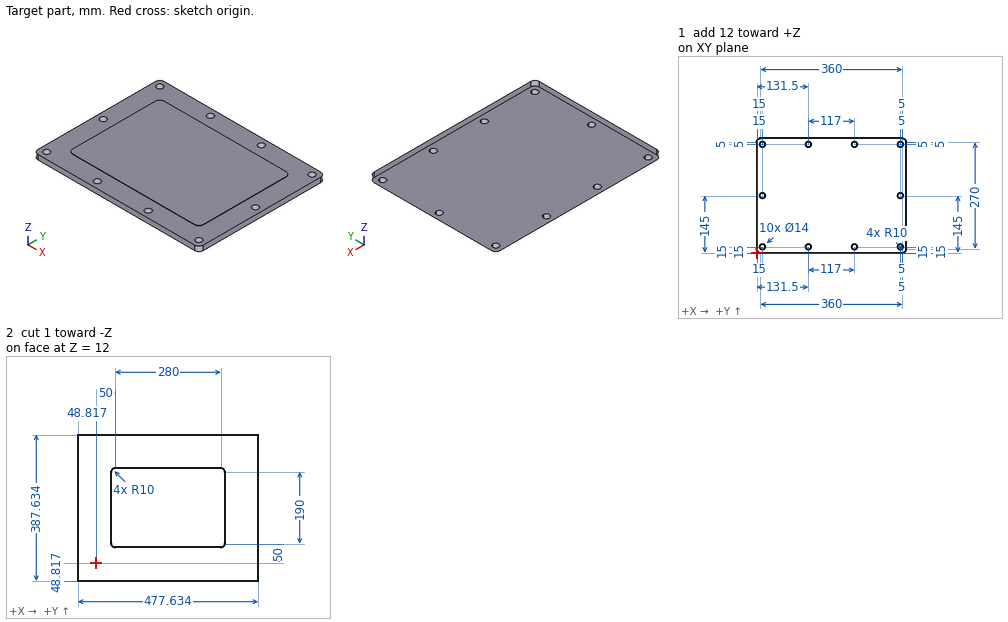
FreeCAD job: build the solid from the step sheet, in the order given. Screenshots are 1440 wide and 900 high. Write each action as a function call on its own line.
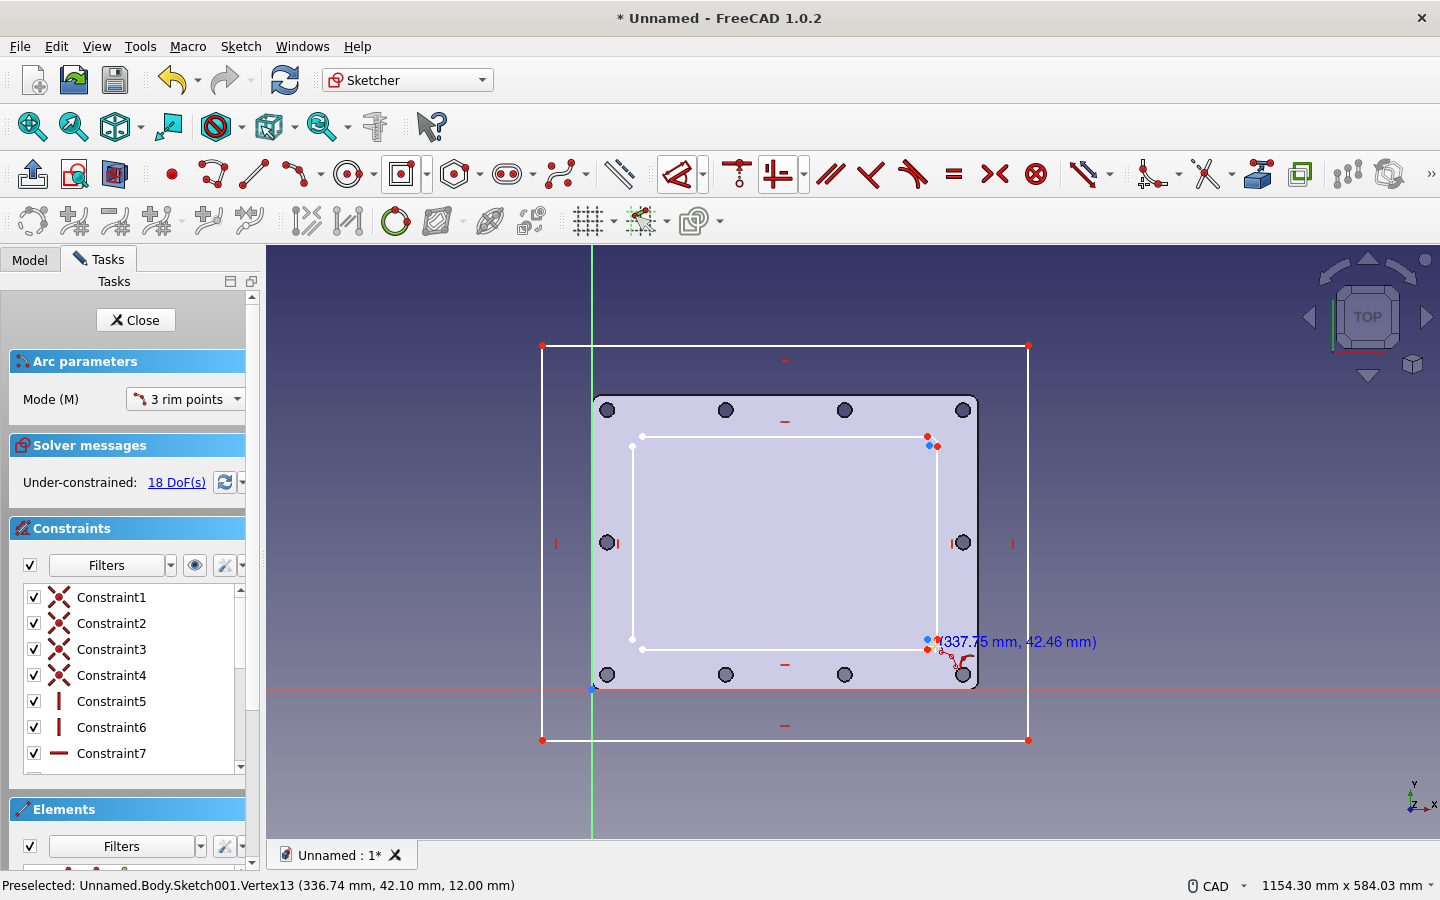
click(643, 650)
click(633, 640)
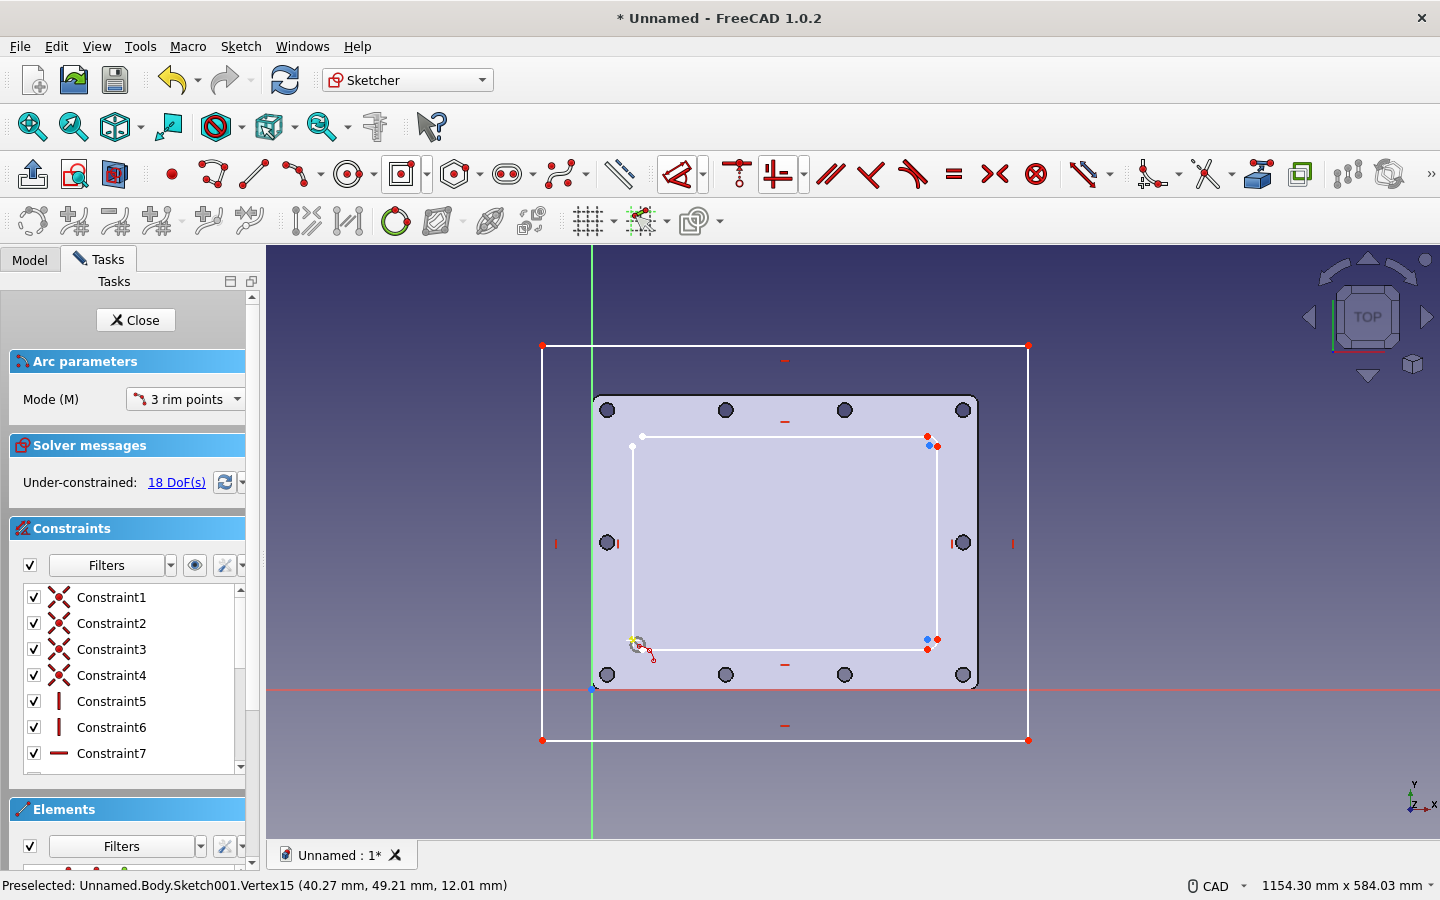
scroll(636, 646, up, 9)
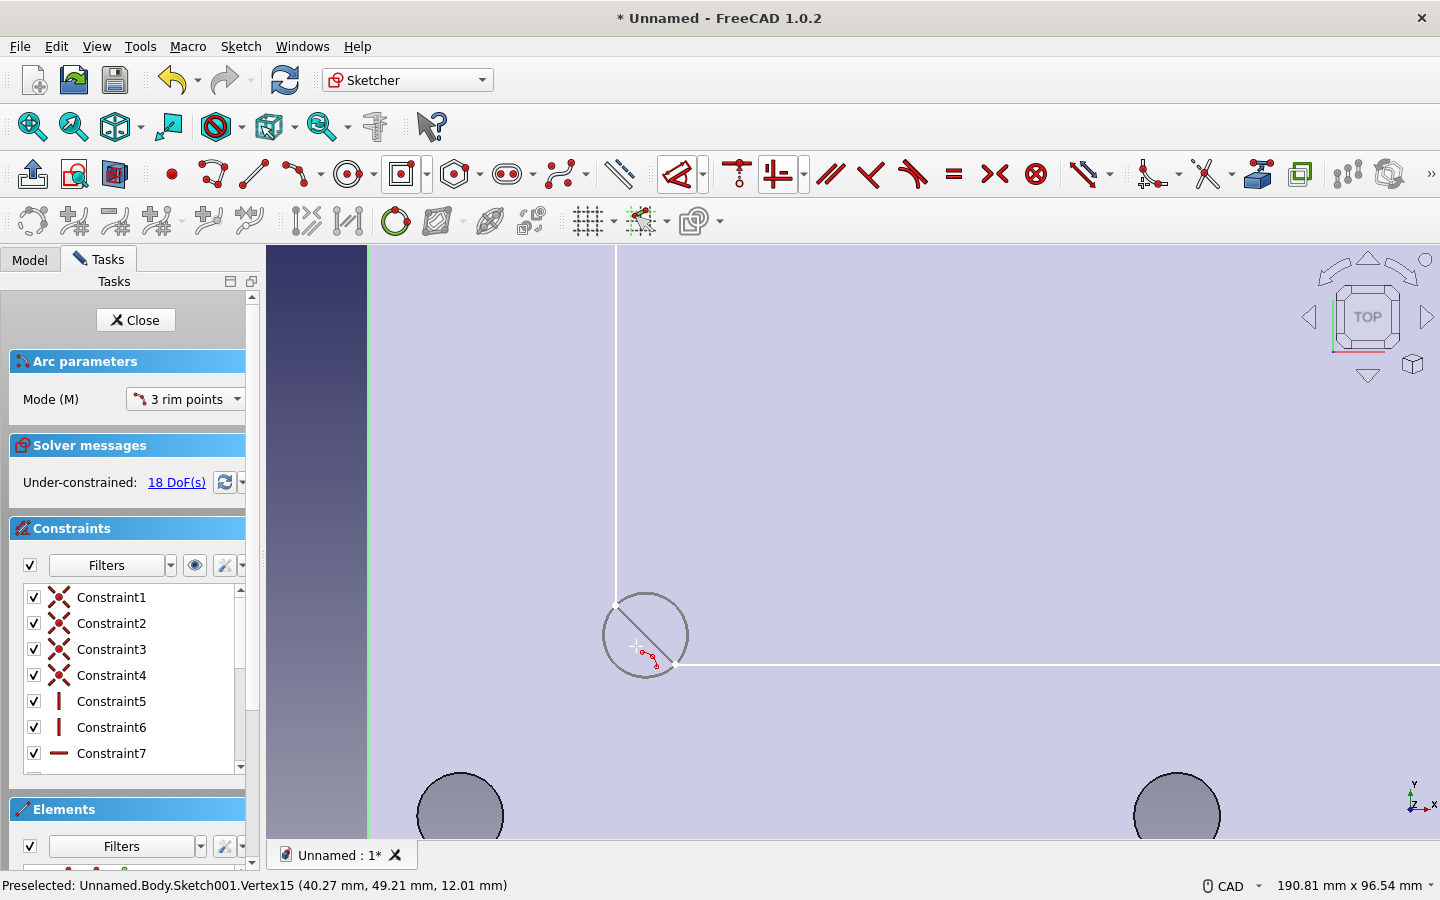
click(632, 644)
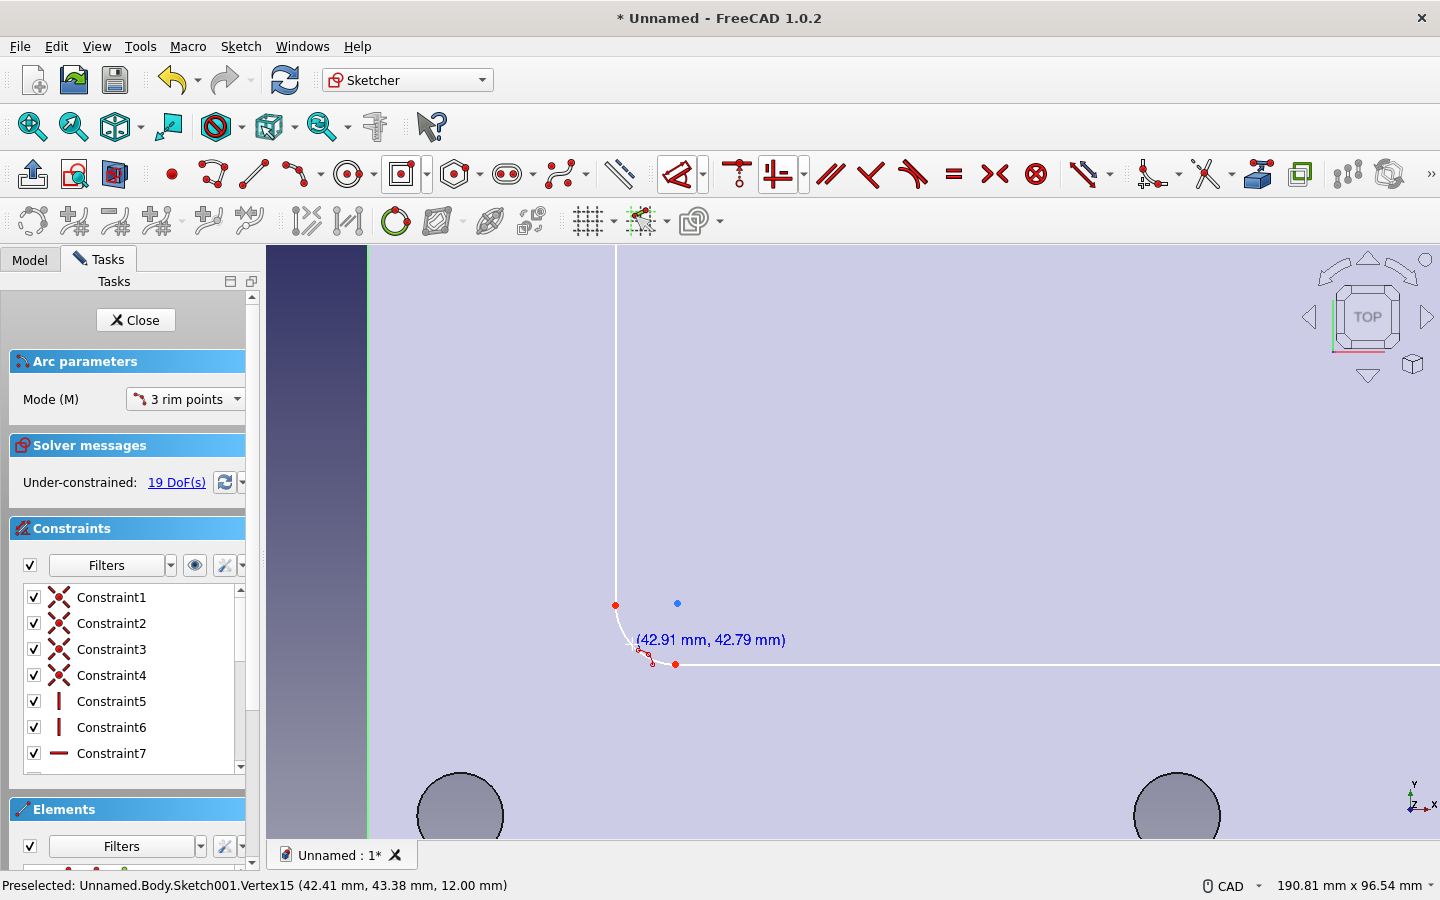
scroll(635, 646, down, 9)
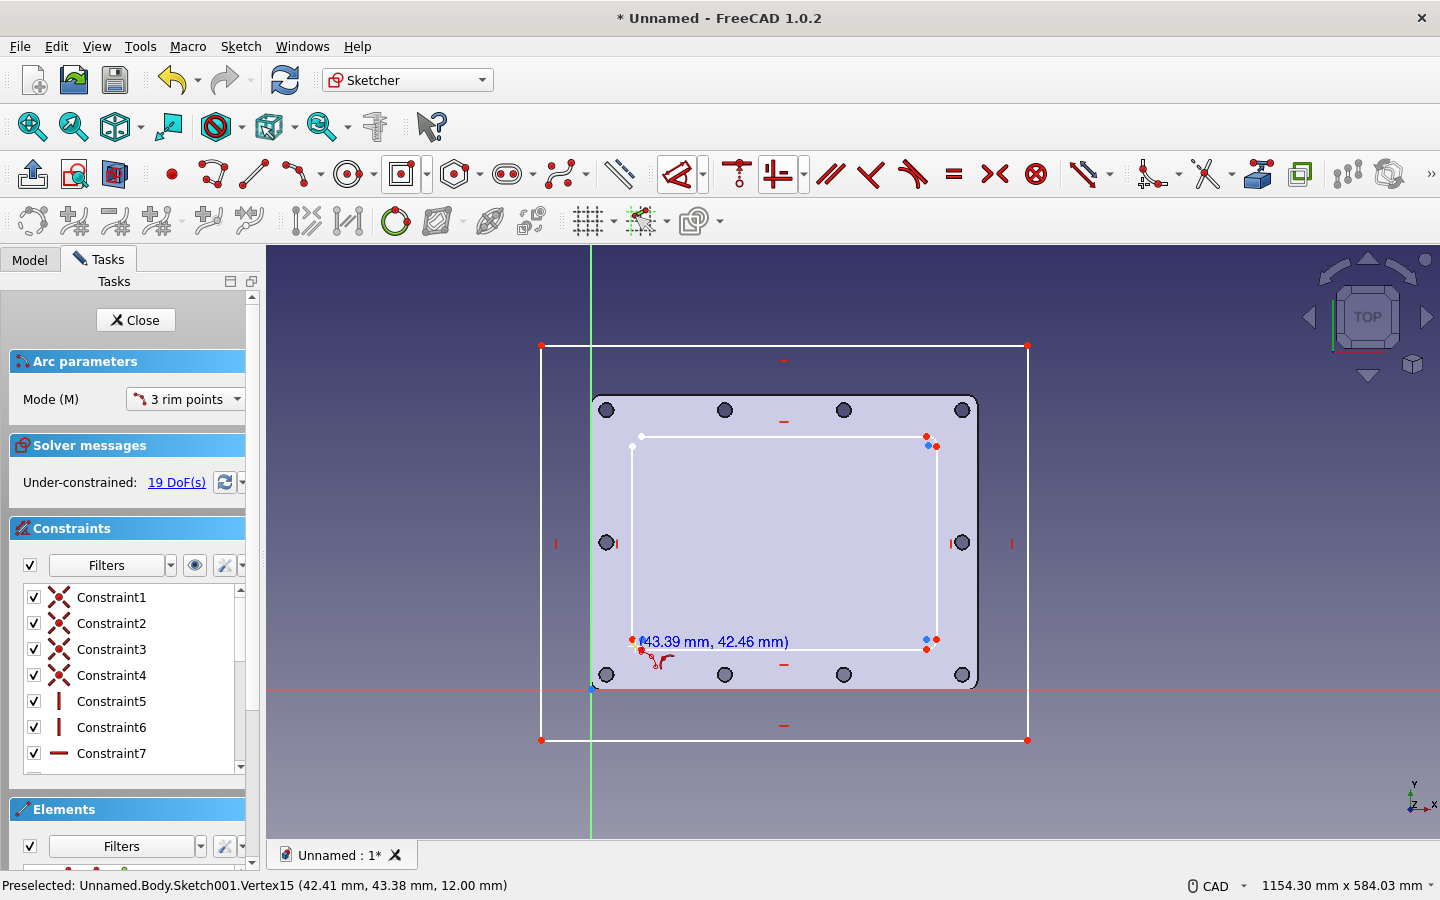
click(632, 447)
click(642, 437)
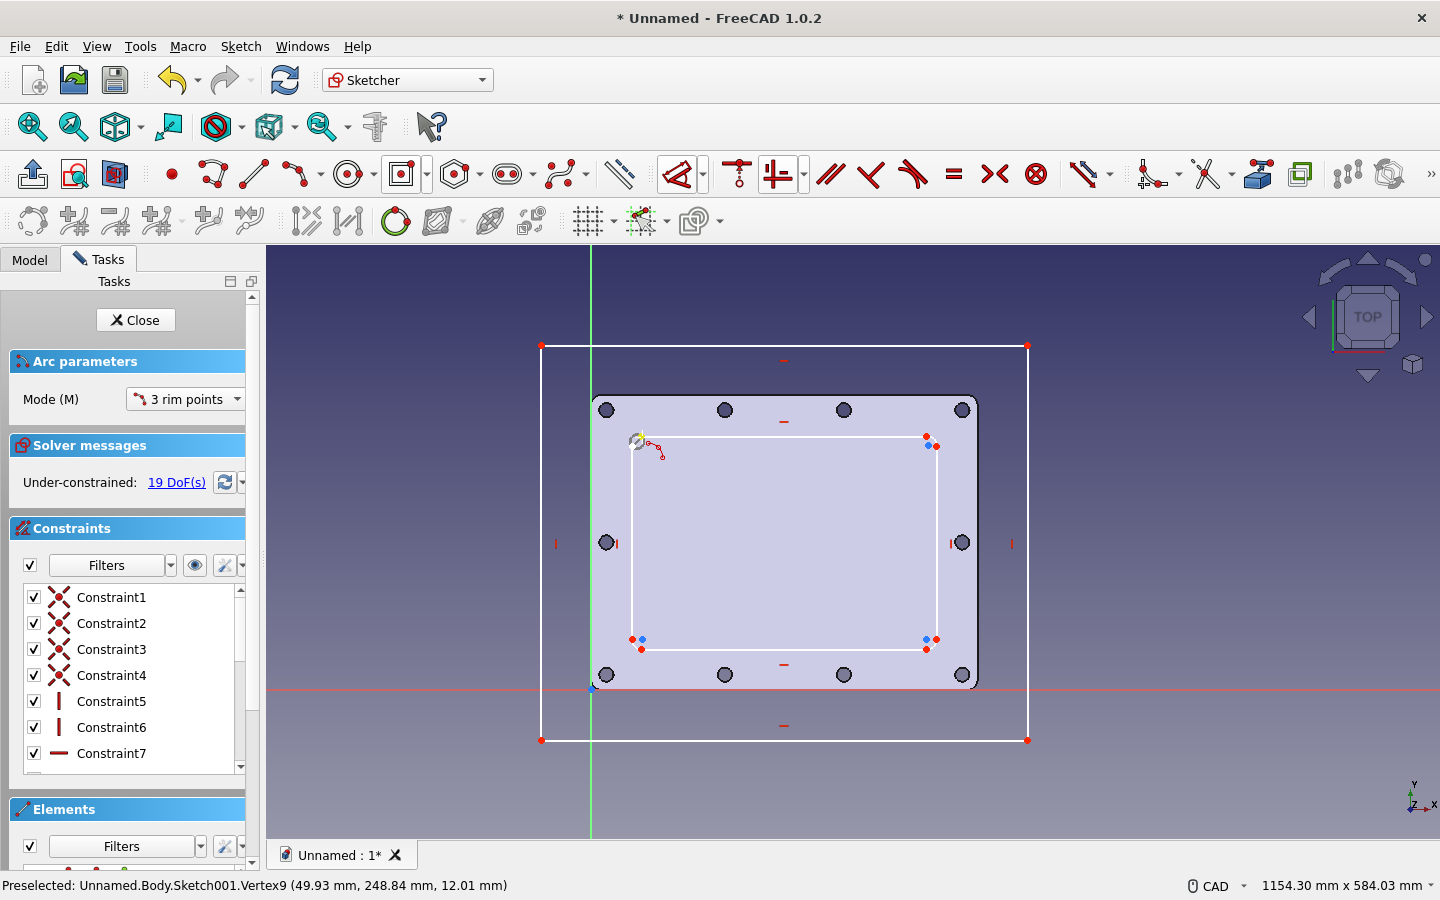
scroll(635, 439, up, 9)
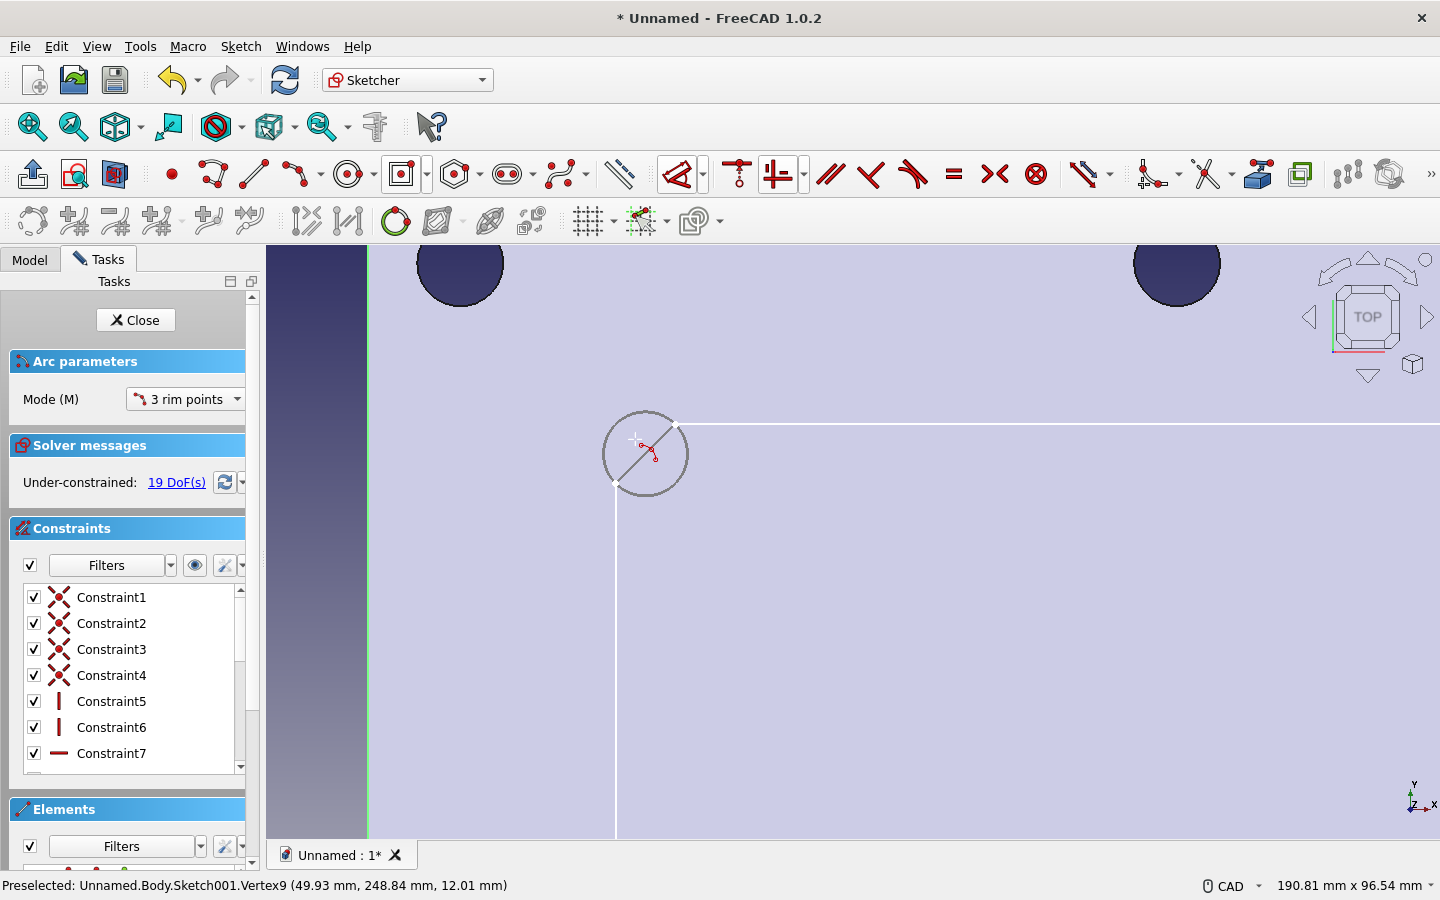
click(632, 435)
key(Escape)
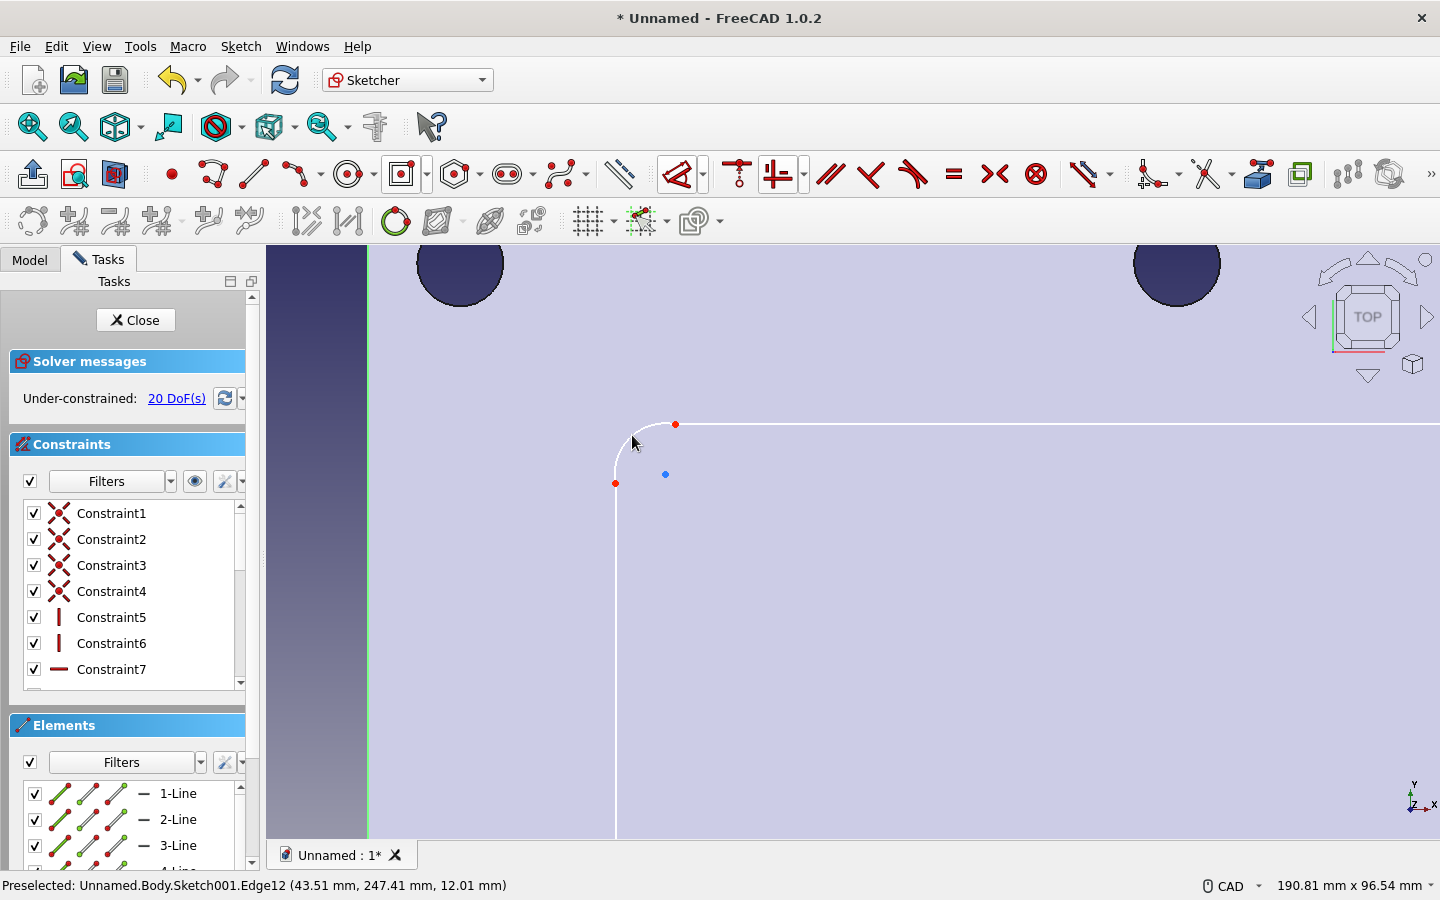
scroll(635, 439, down, 9)